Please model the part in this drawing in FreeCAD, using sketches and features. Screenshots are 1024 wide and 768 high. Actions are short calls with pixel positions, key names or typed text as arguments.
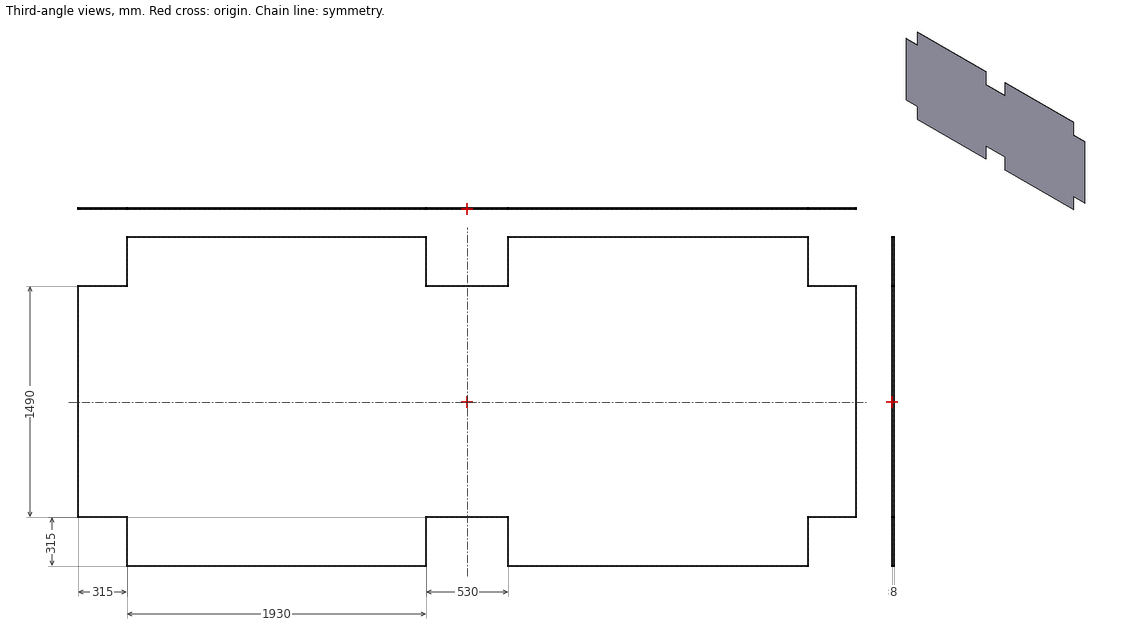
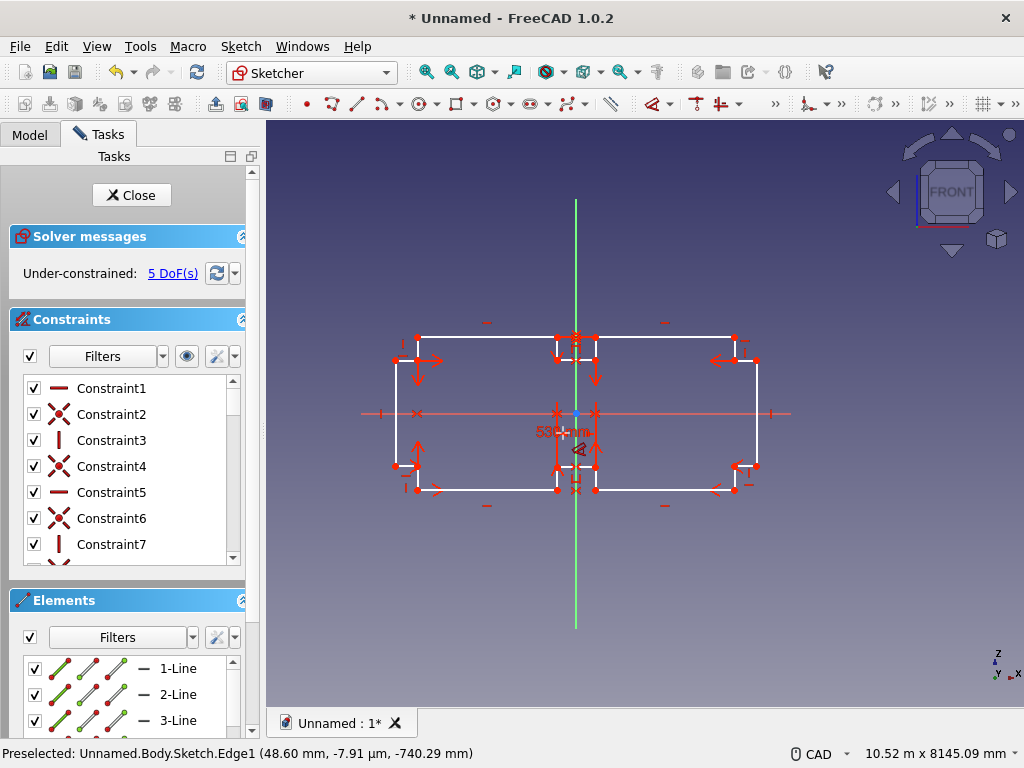
scroll(557, 476, up, 3)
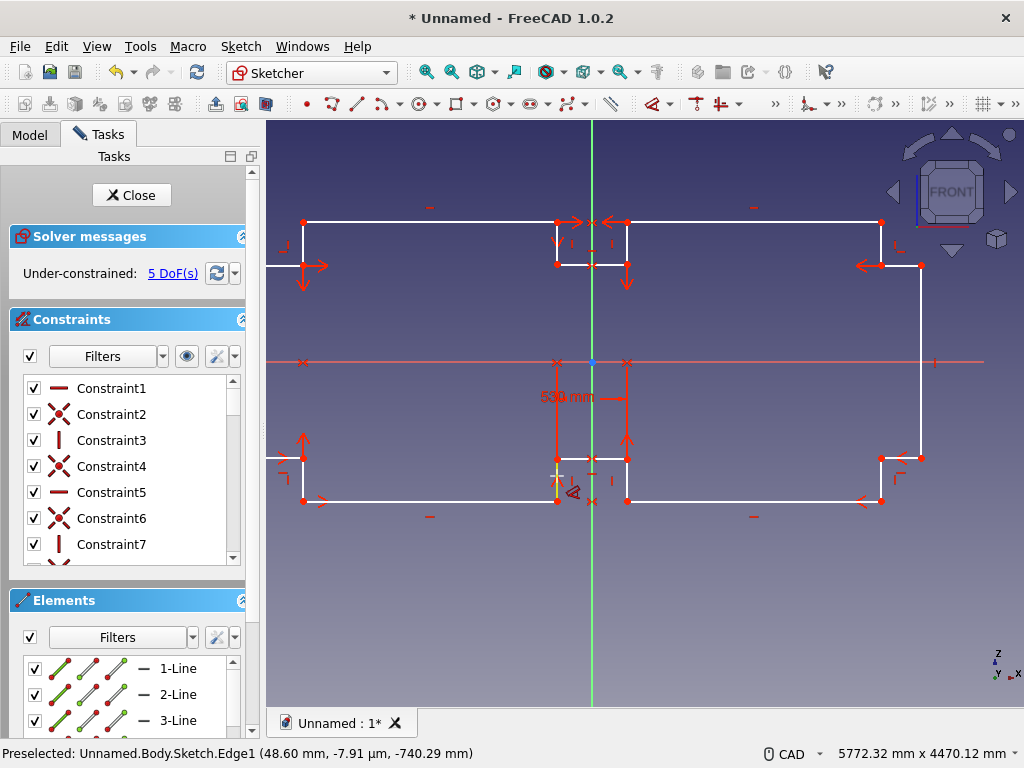
click(557, 476)
click(523, 480)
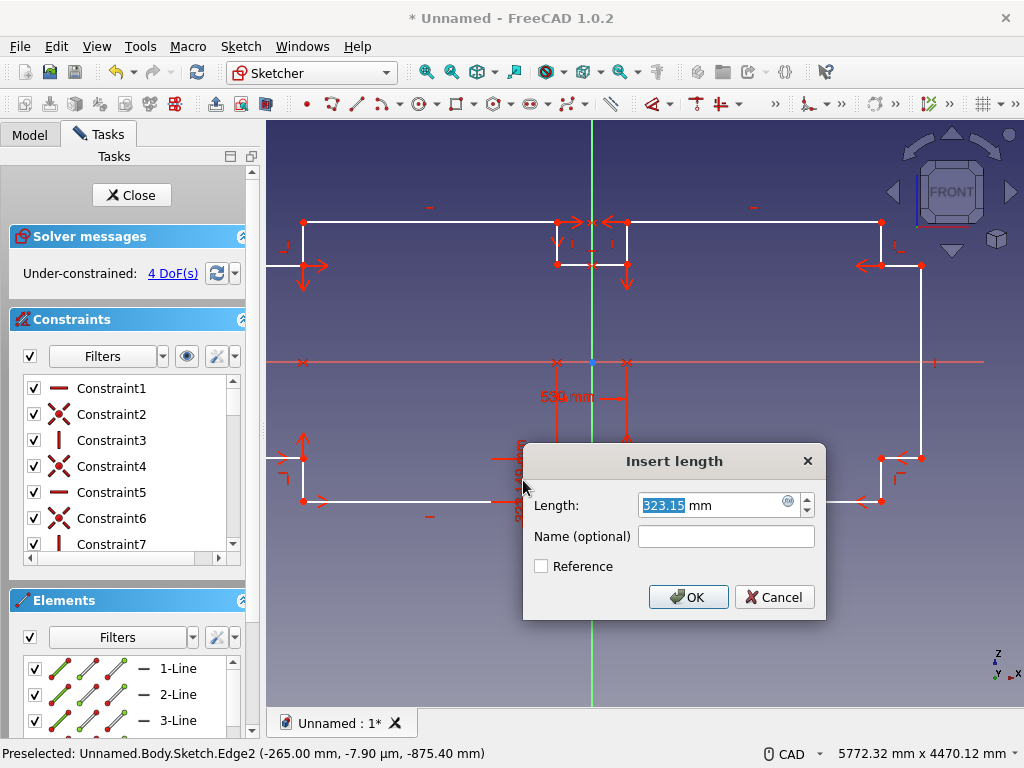
text(315)
key(Return)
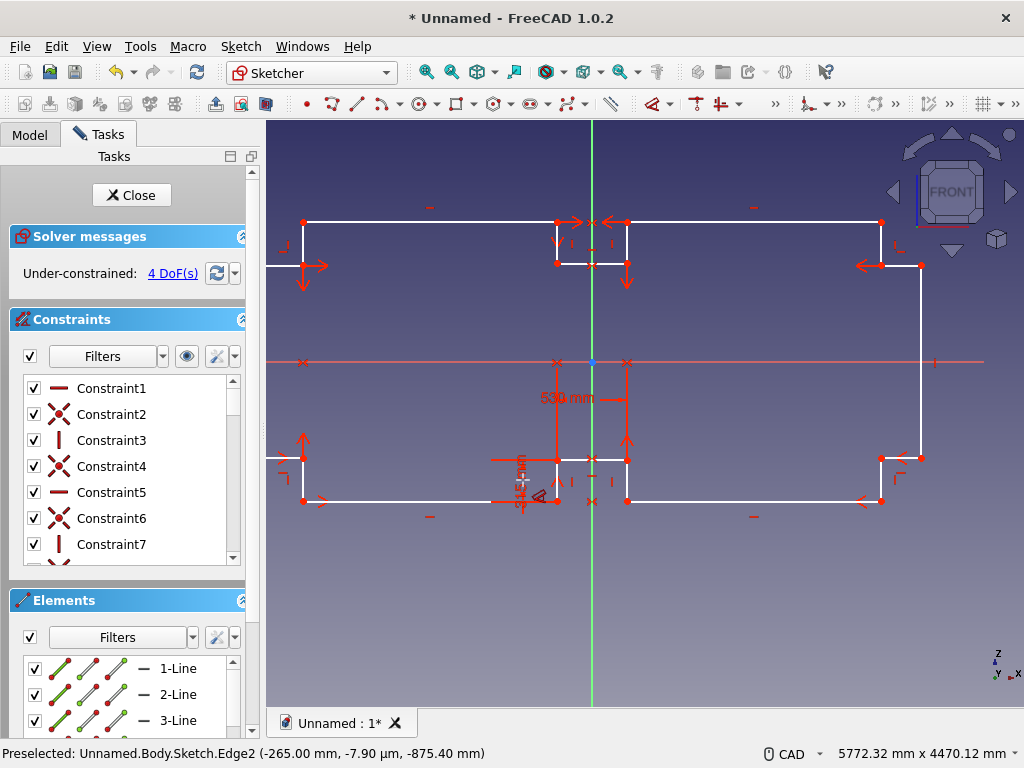
click(303, 489)
click(337, 480)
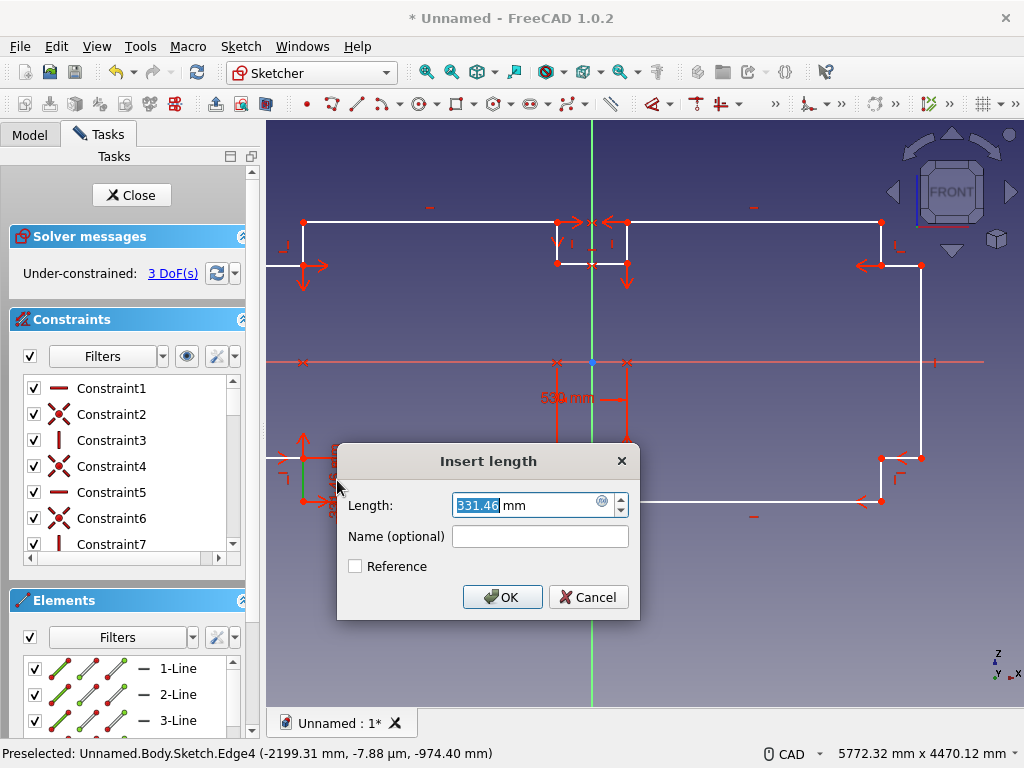
text(315)
key(Return)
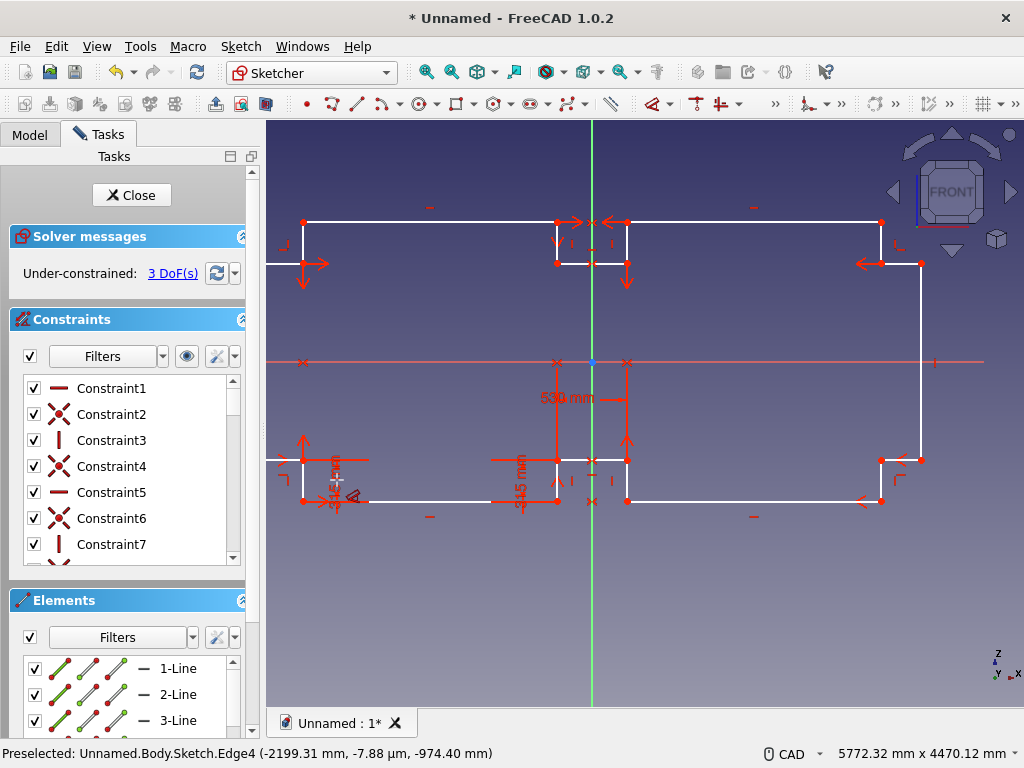
scroll(557, 476, down, 3)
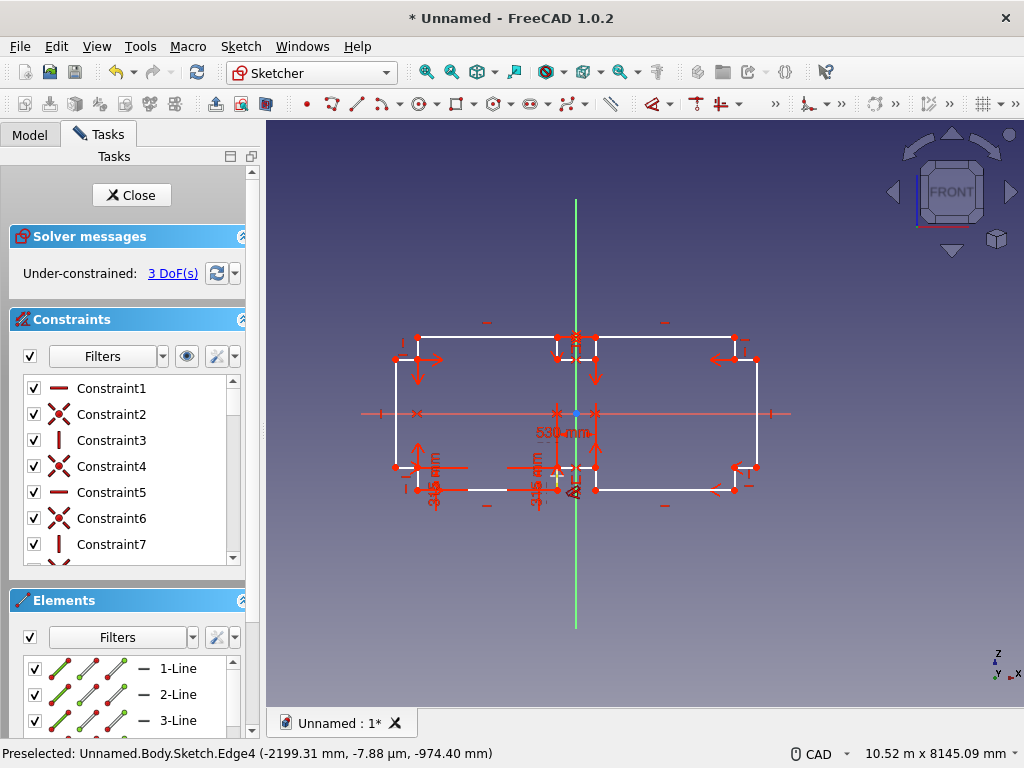
scroll(411, 468, up, 4)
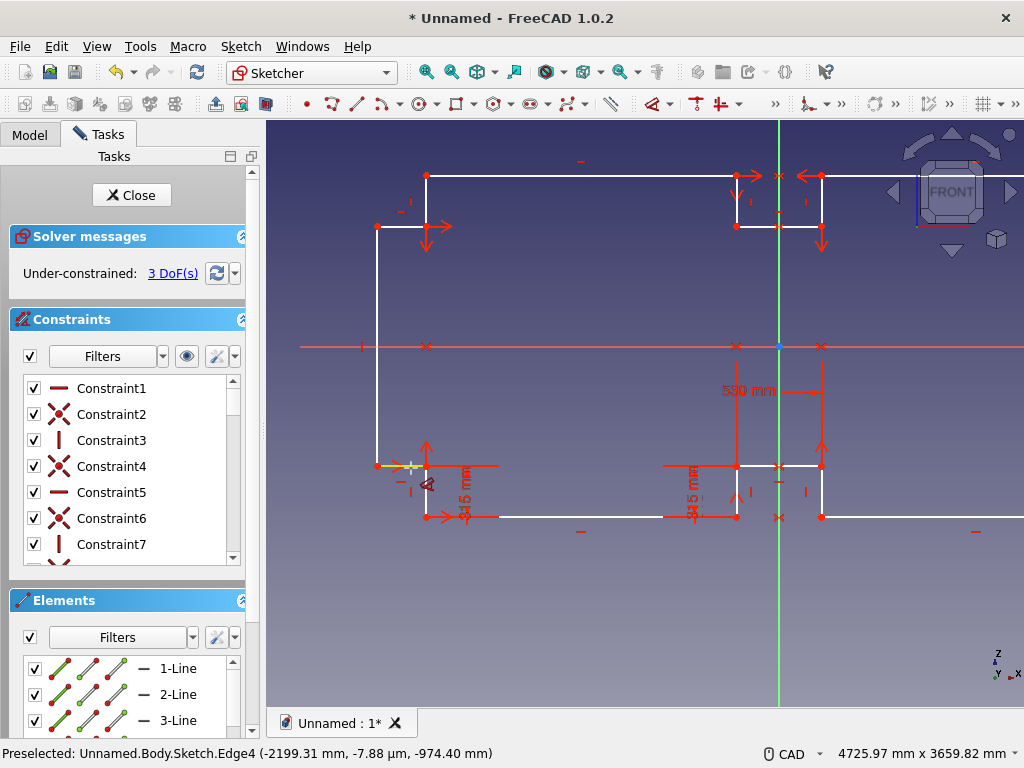
click(412, 466)
click(391, 500)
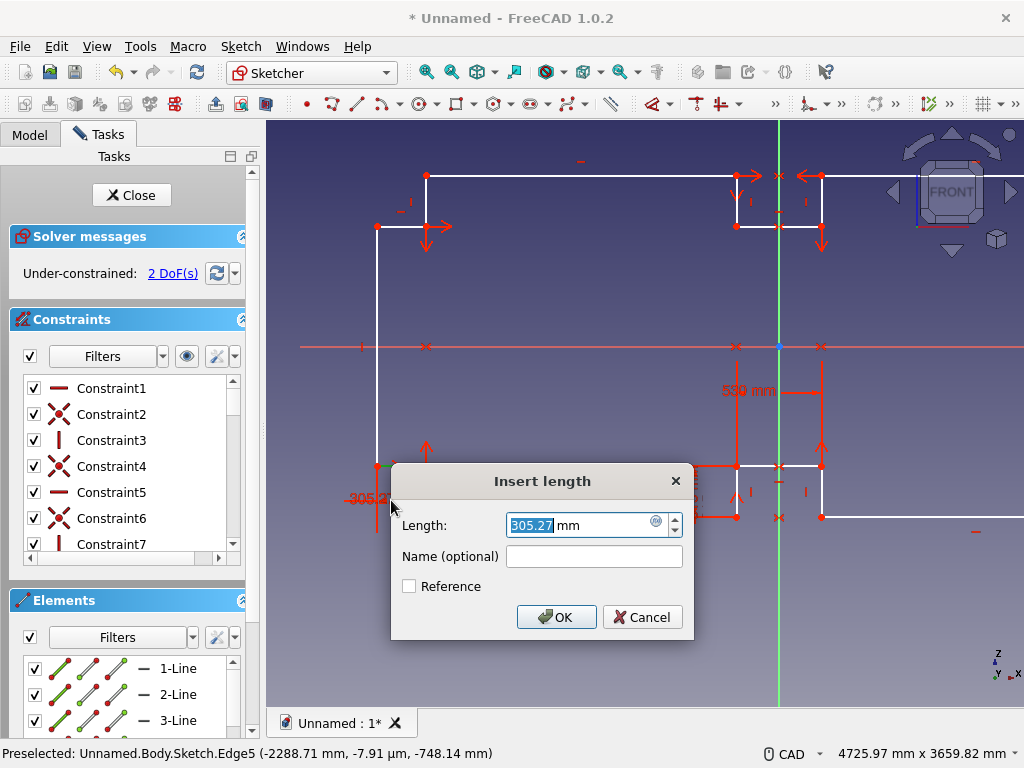
text(315)
key(Return)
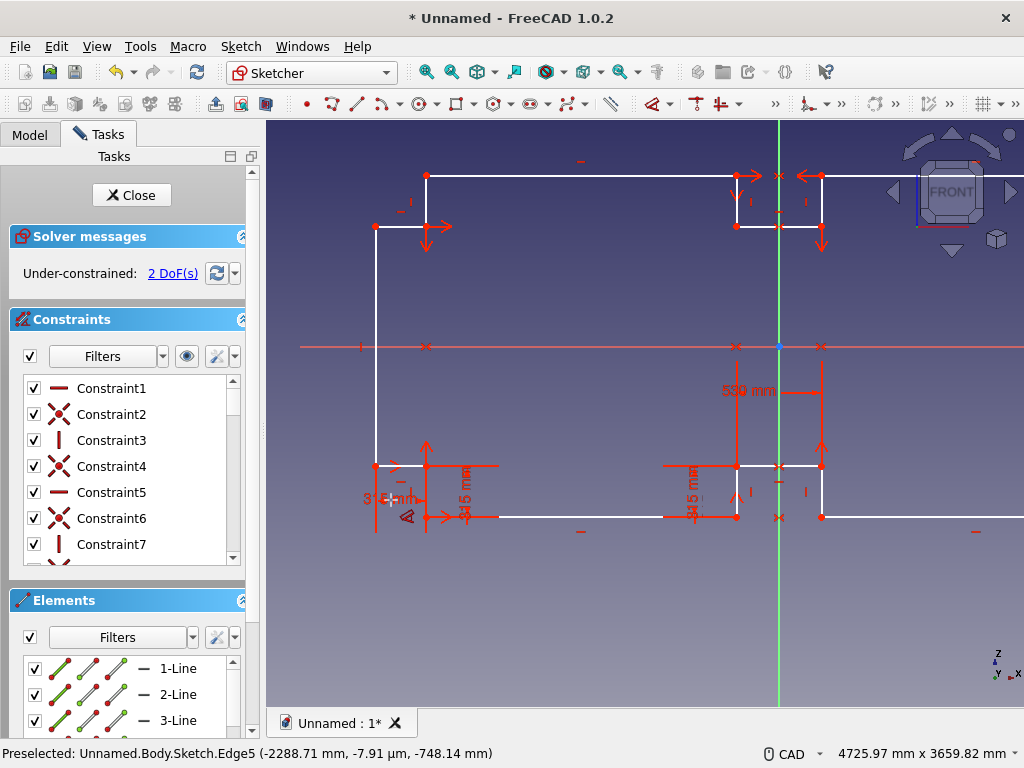
click(644, 517)
click(581, 551)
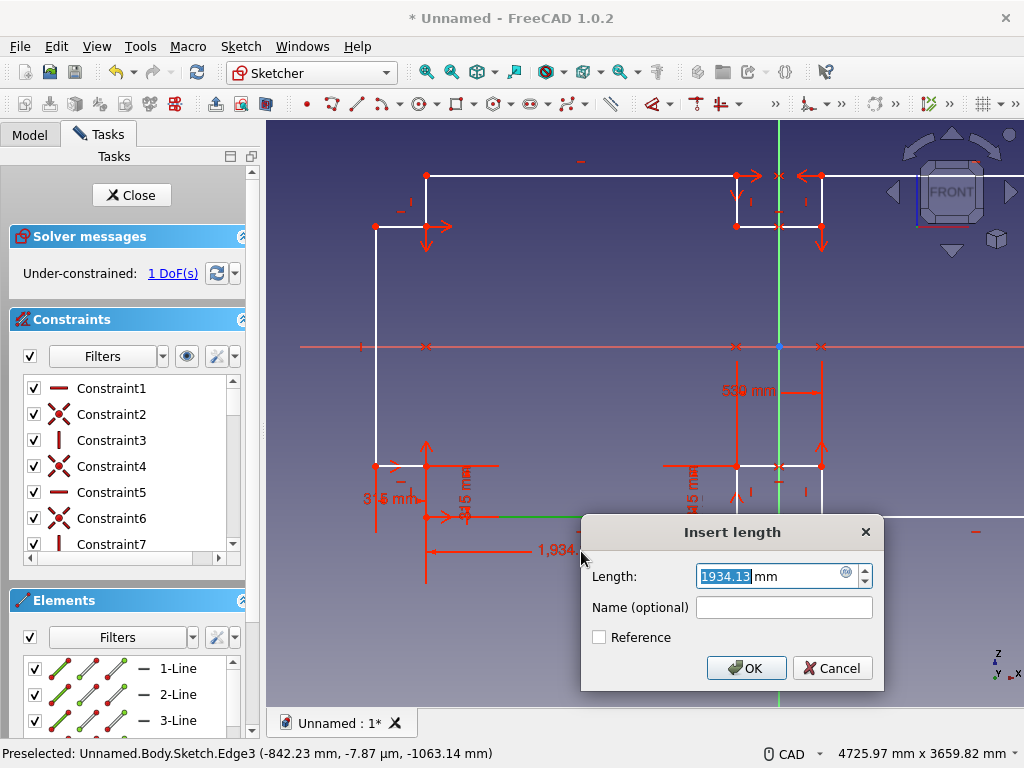
text(1930)
key(Return)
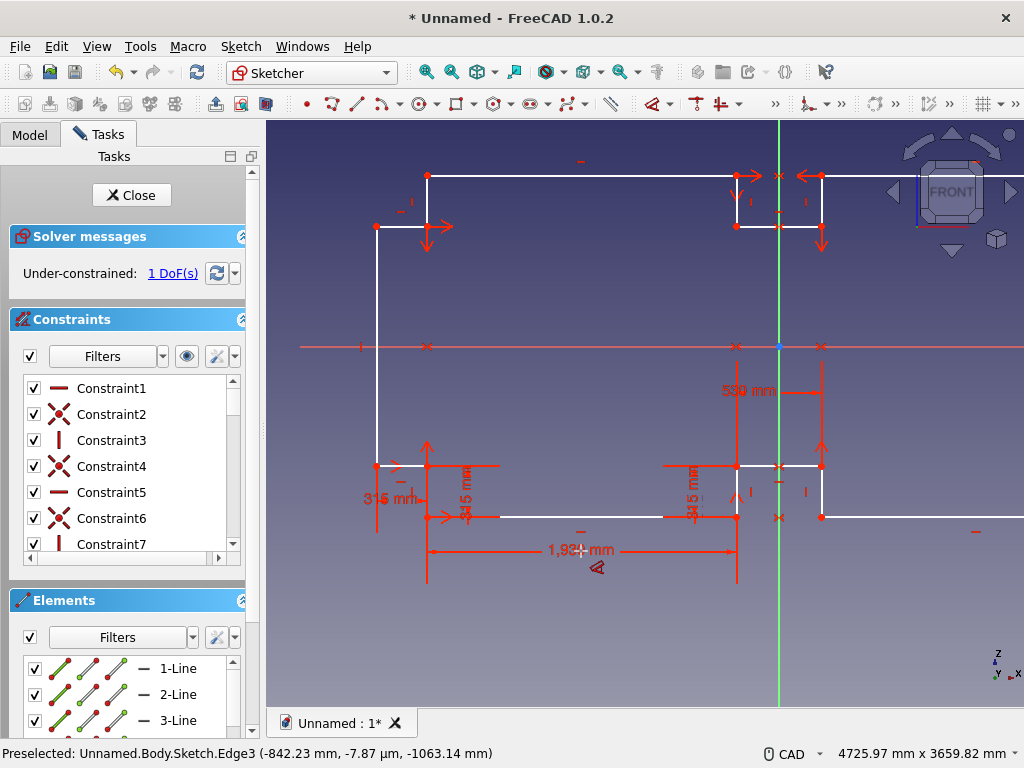
click(377, 395)
click(343, 291)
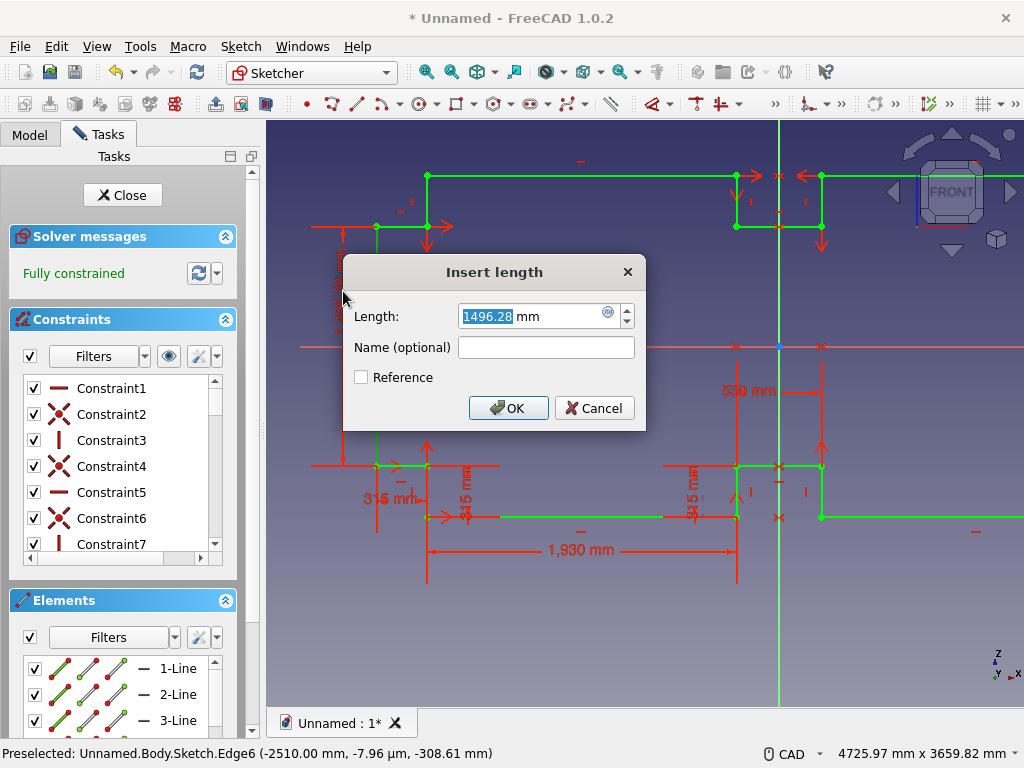
text(1490)
key(Return)
key(Escape)